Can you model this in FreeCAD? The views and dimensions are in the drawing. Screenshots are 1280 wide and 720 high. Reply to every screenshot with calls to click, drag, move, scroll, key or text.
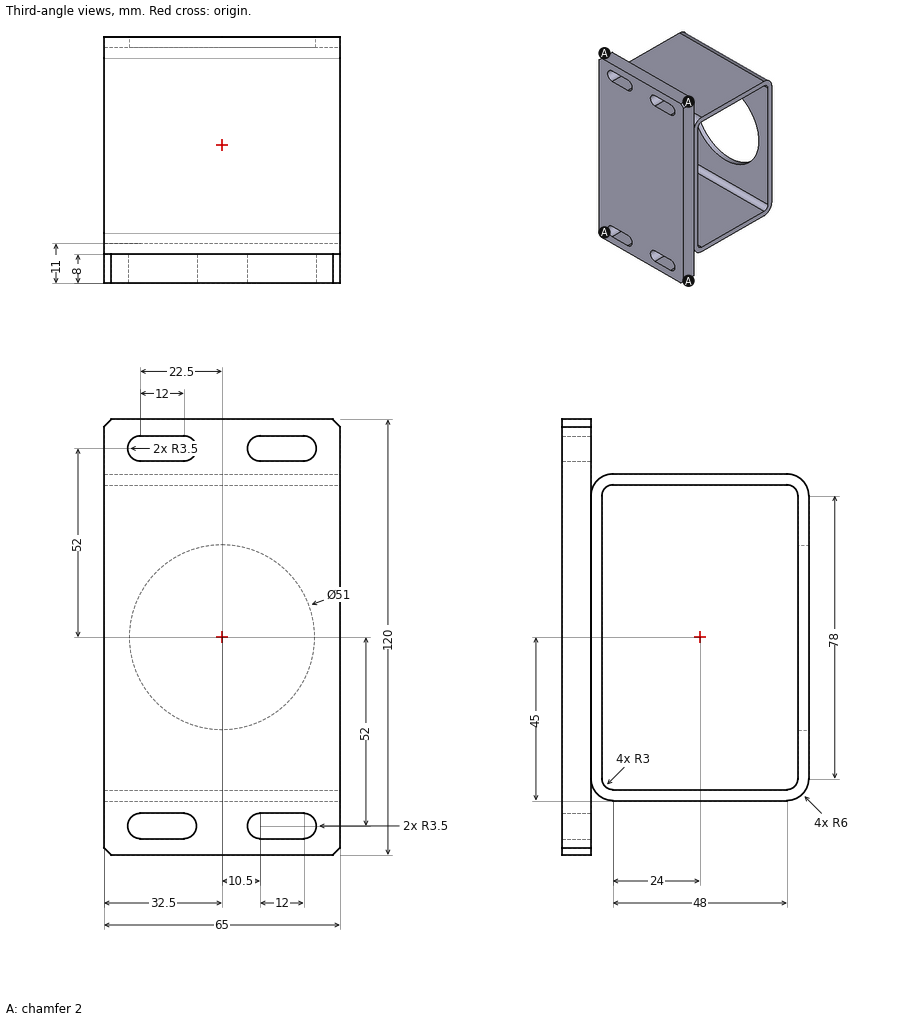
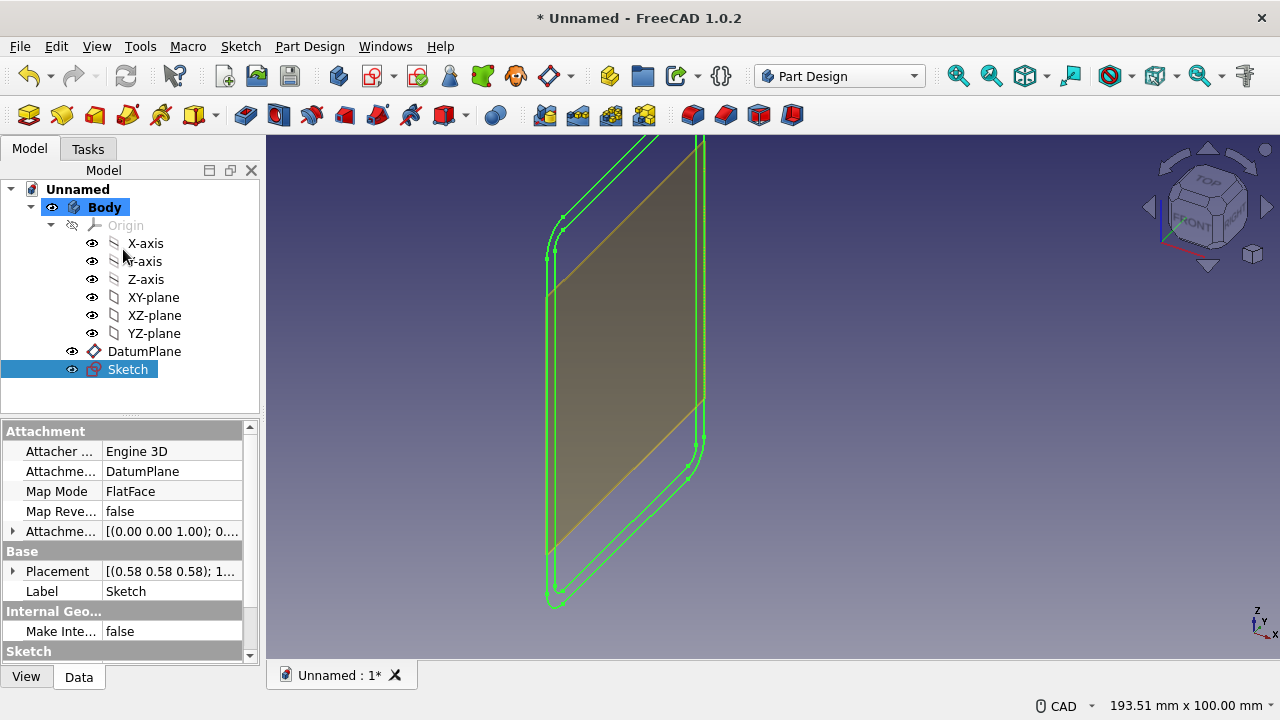
click(29, 116)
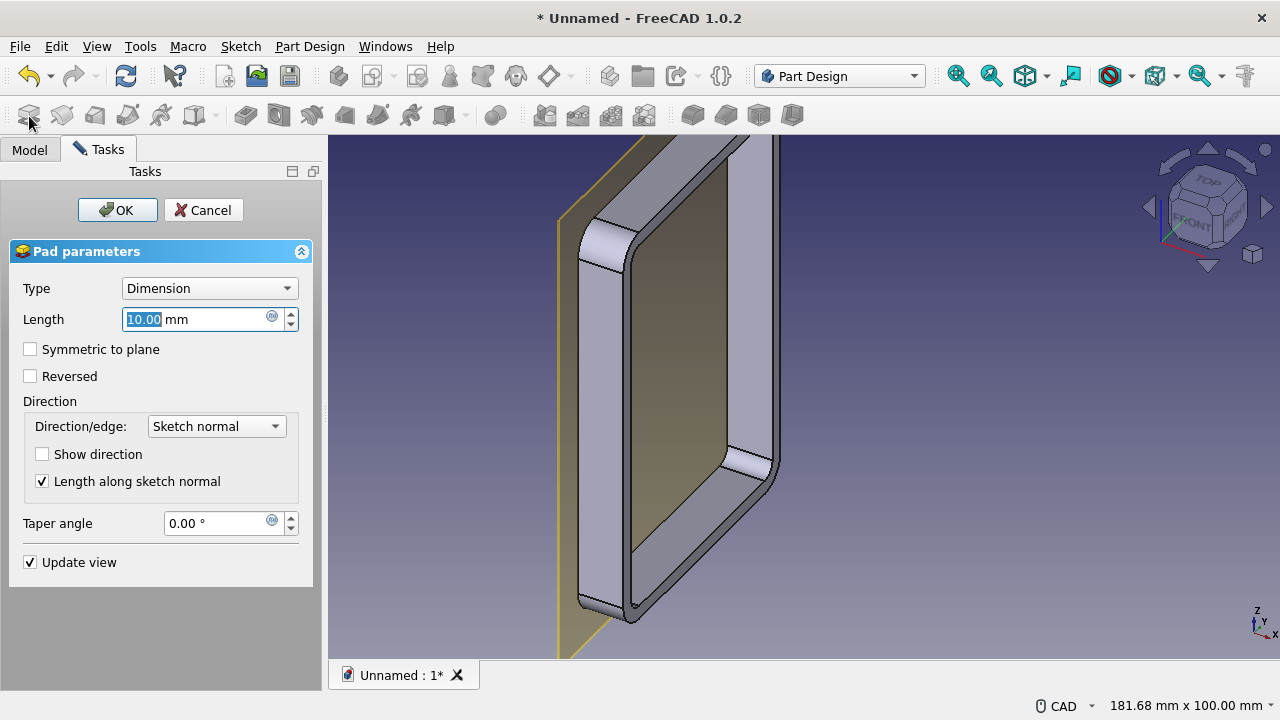
text(65)
key(Tab)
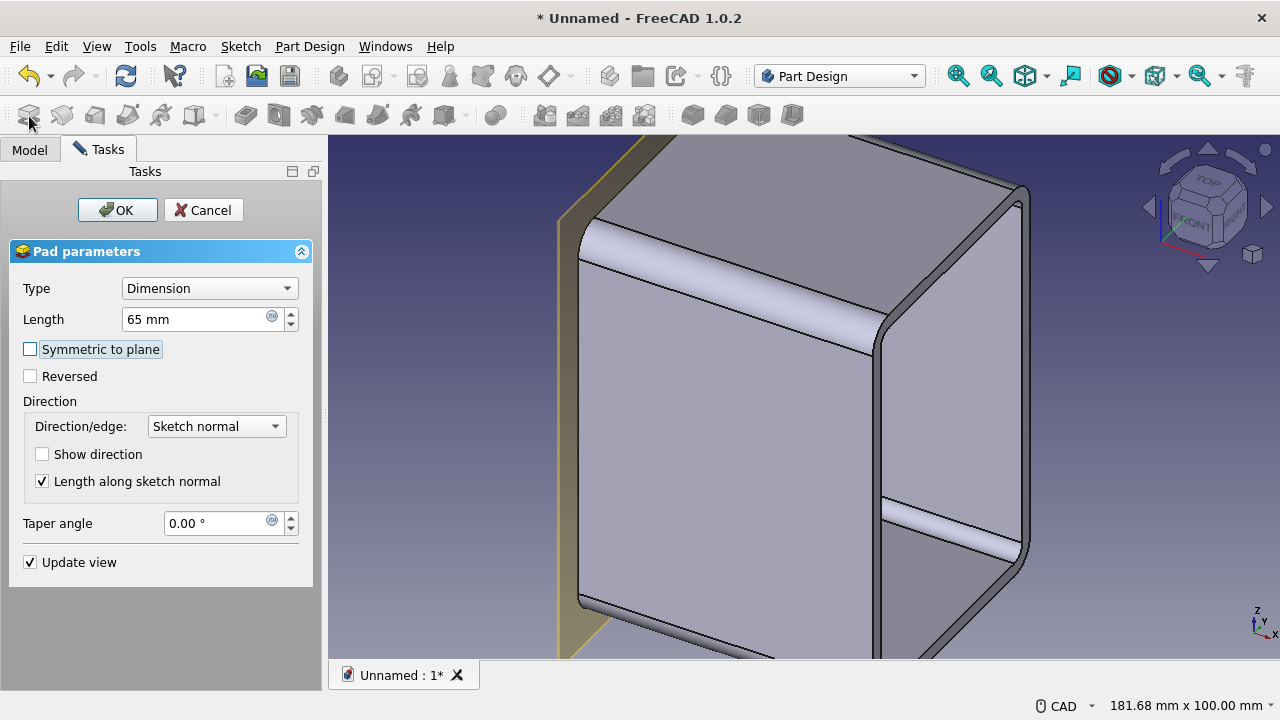
click(118, 210)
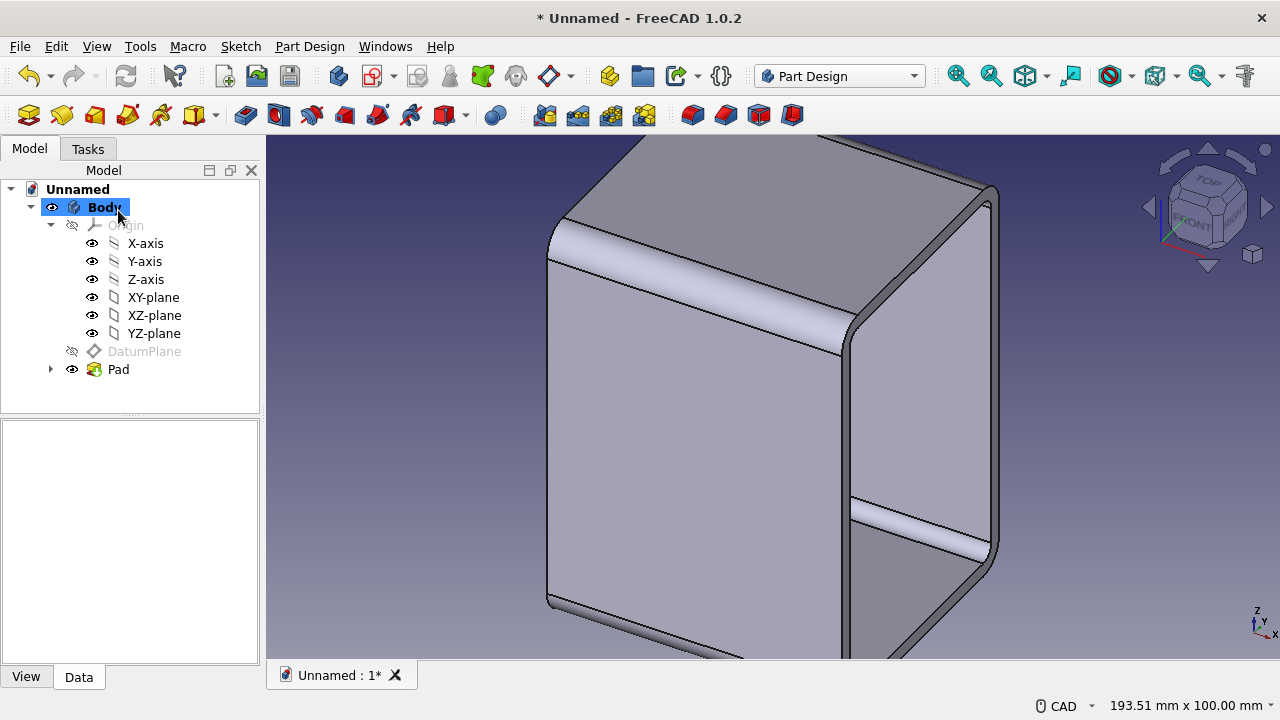
click(959, 76)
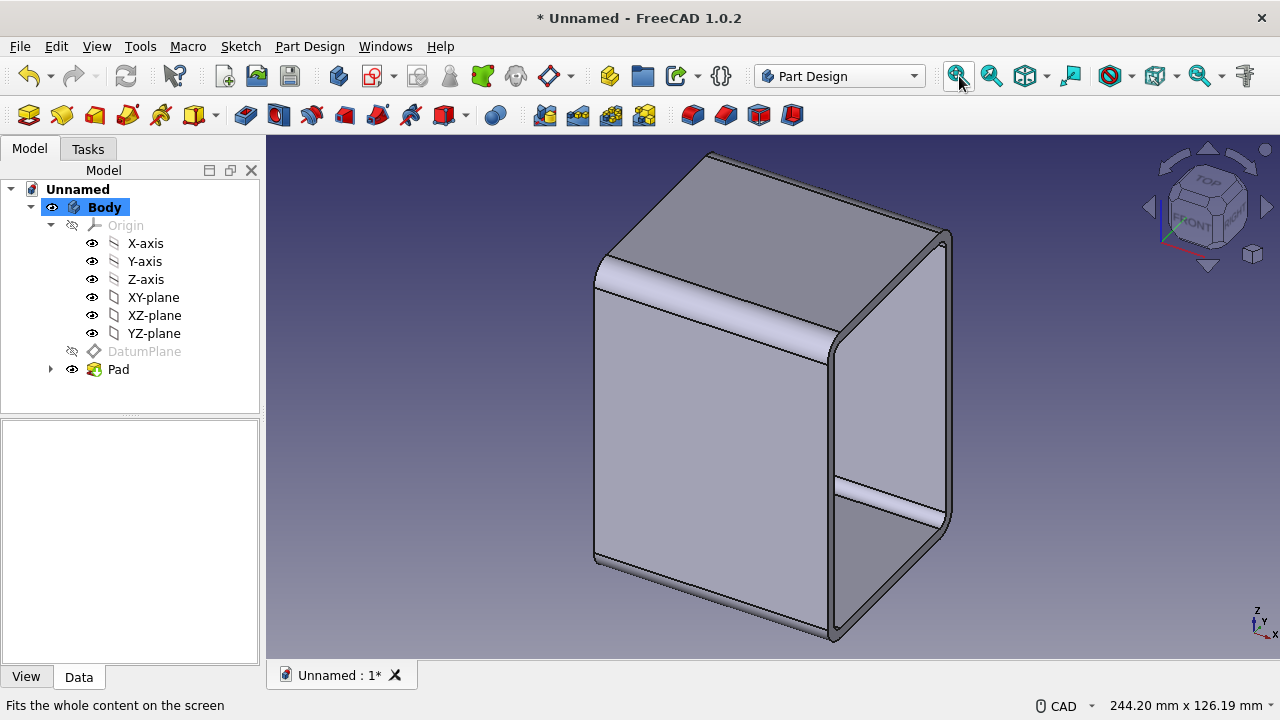
key(4)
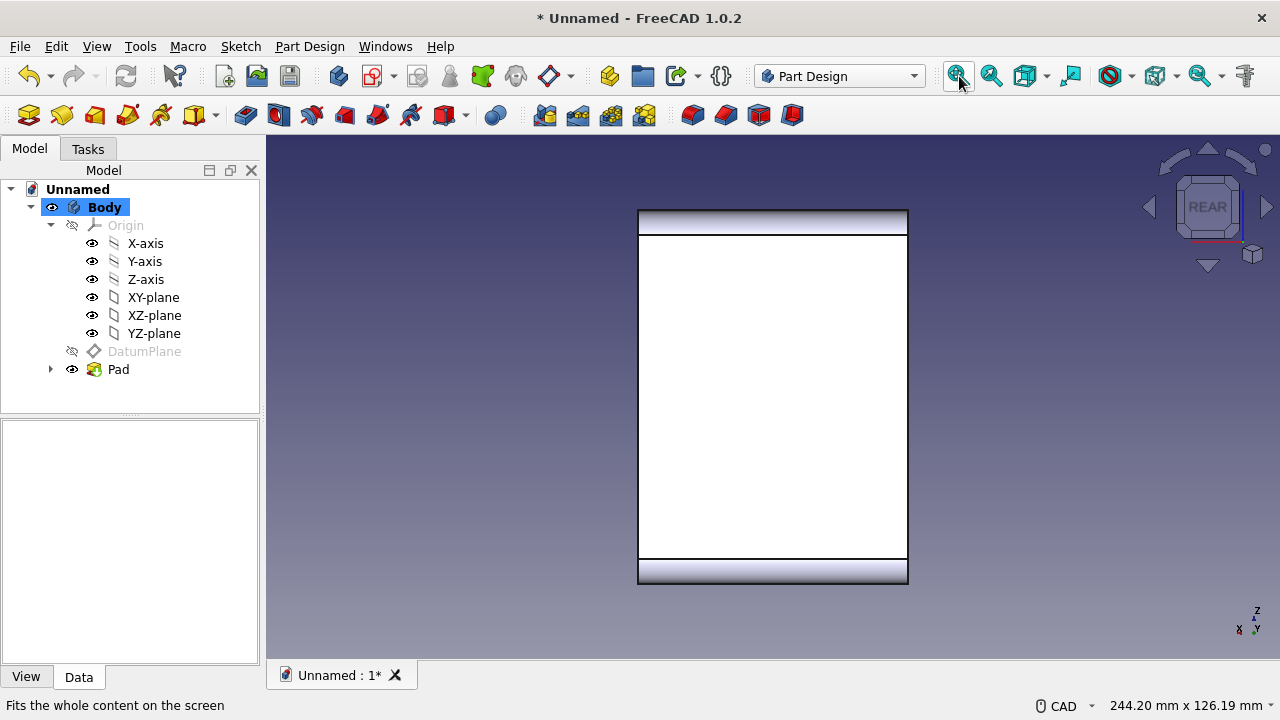
click(773, 396)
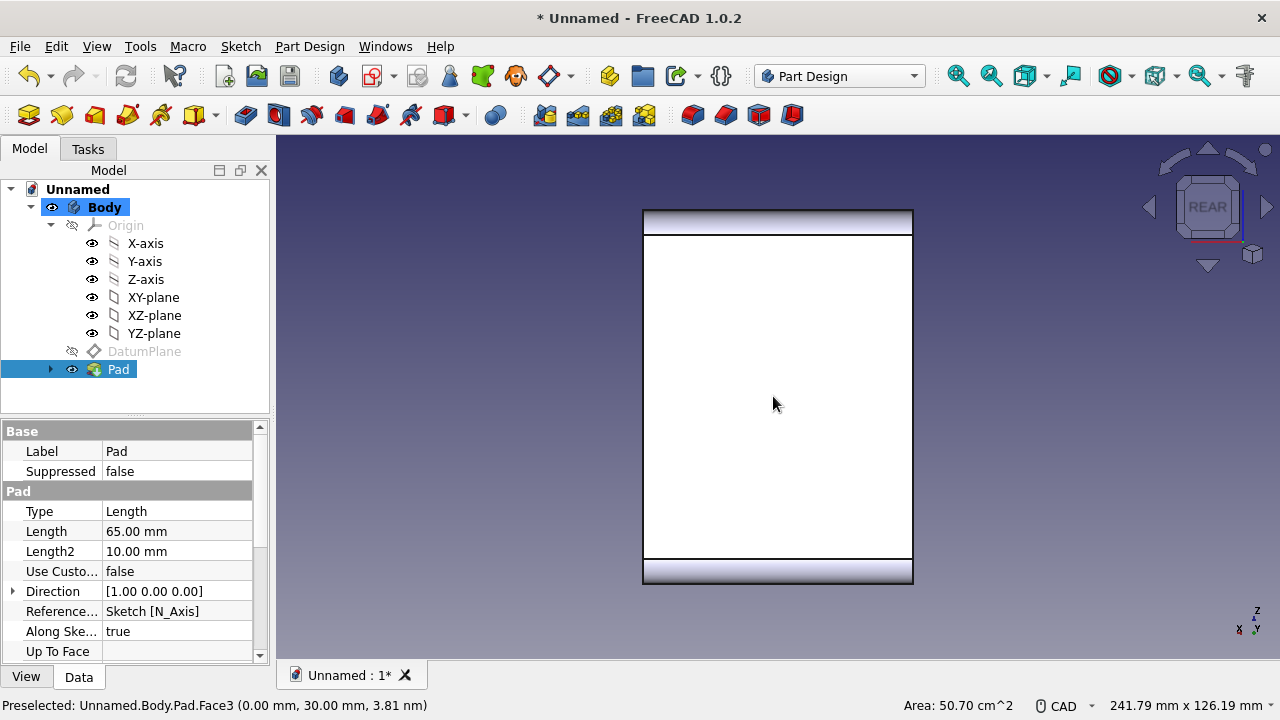
click(372, 76)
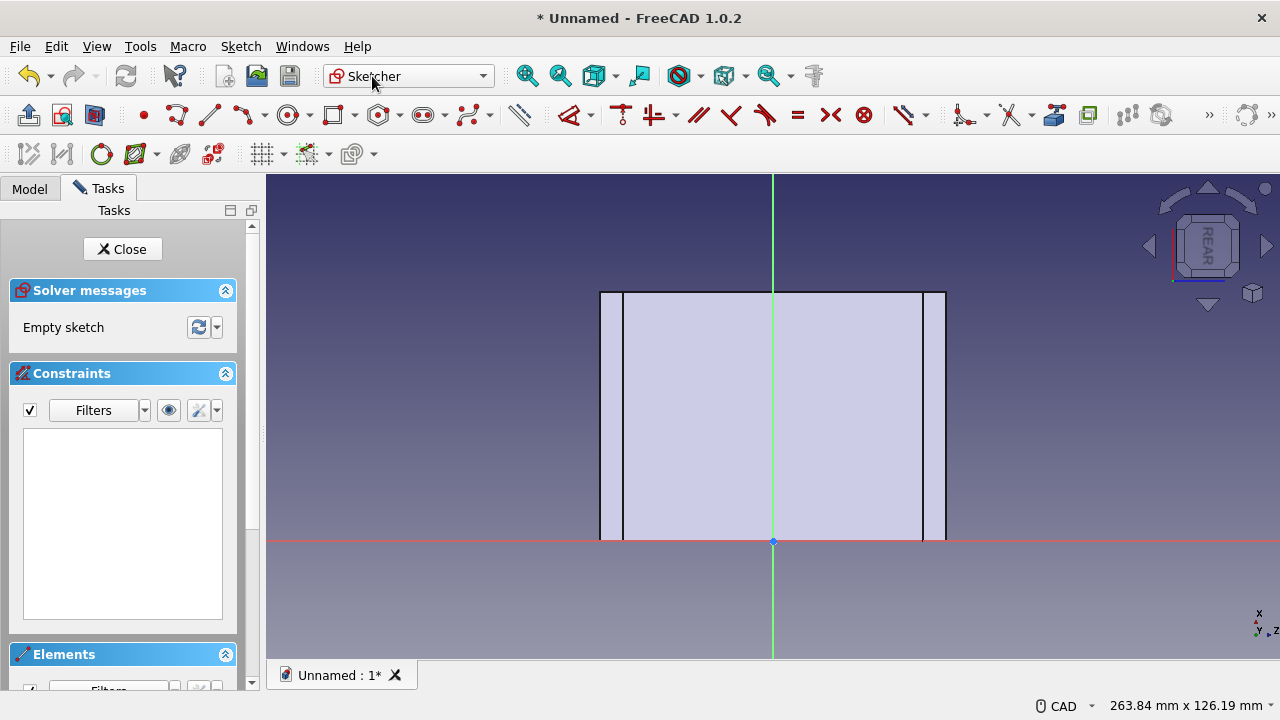
scroll(912, 457, up, 2)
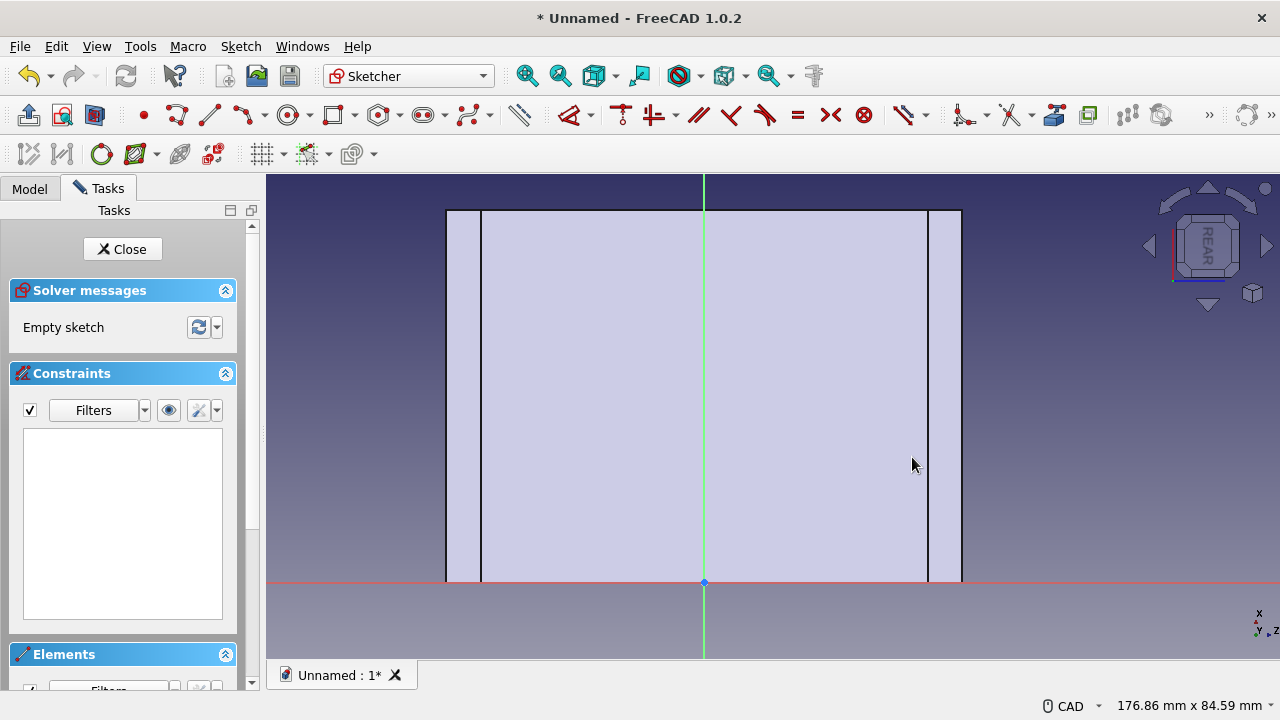
click(288, 116)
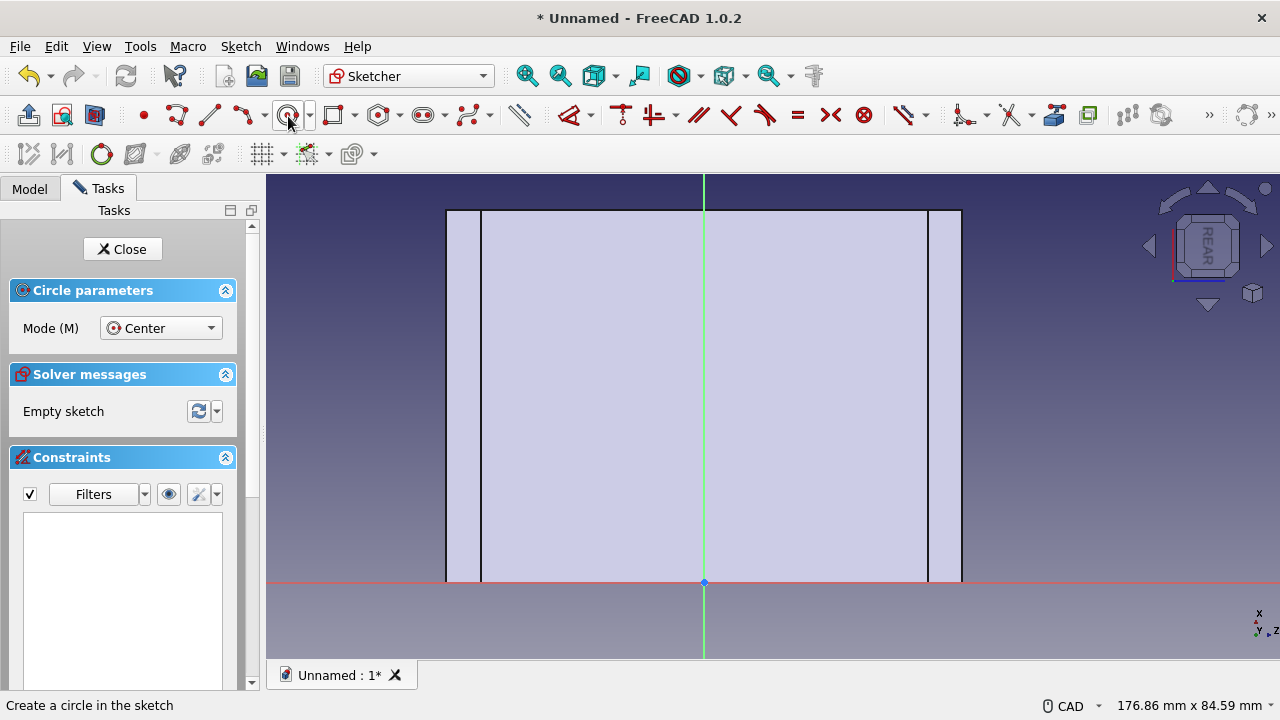
click(704, 396)
move(808, 293)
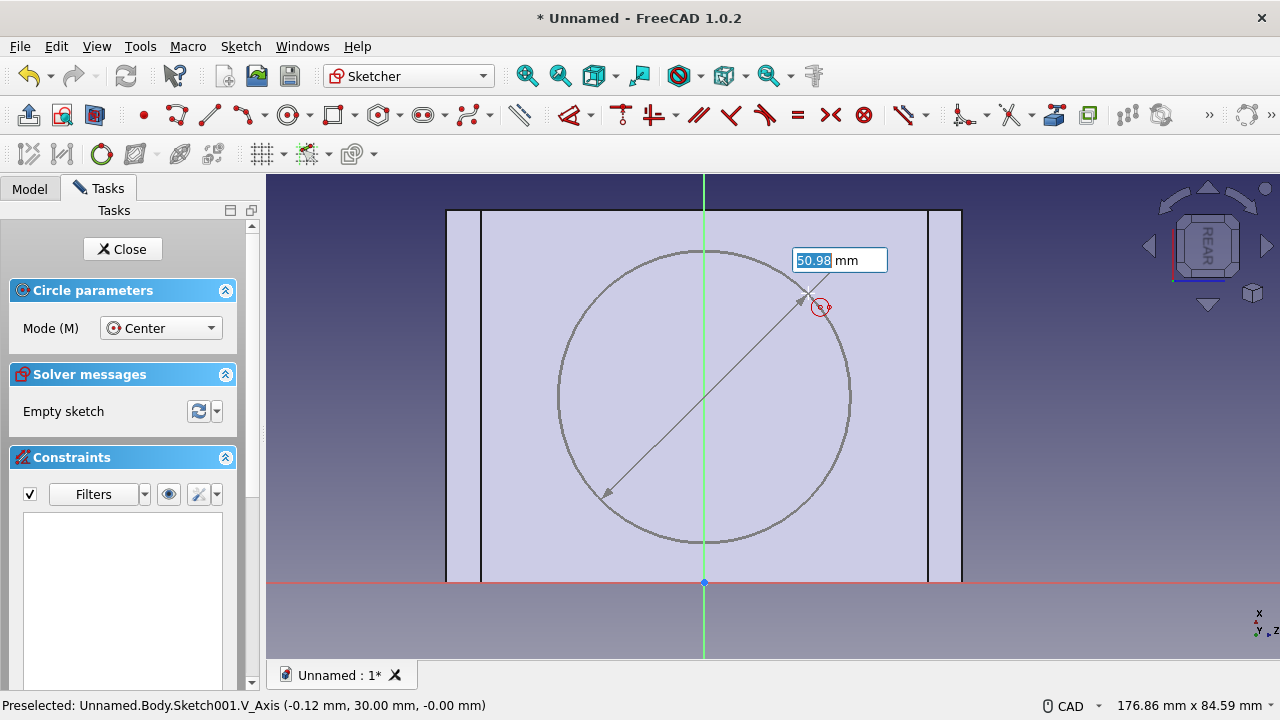
text(51)
key(Return)
key(Escape)